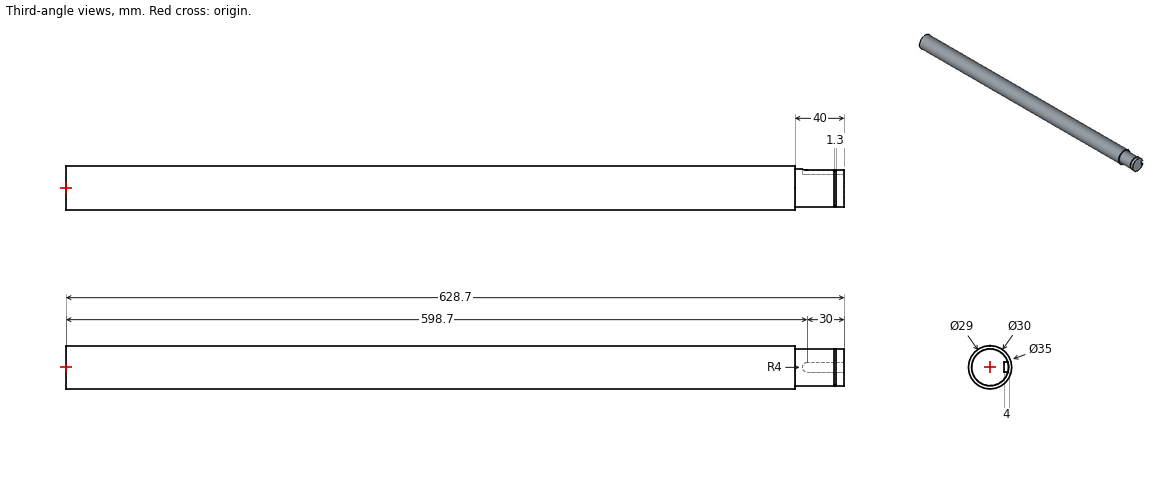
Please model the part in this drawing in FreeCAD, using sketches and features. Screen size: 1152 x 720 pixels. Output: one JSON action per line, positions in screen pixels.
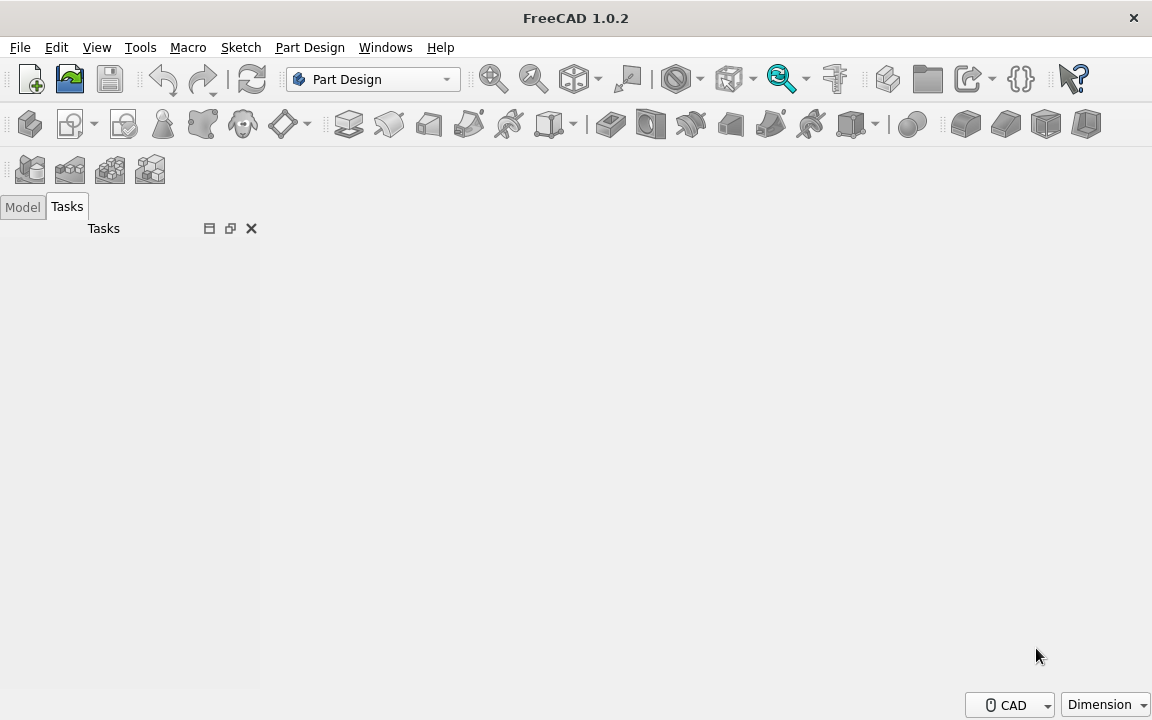
{"action": "left_click", "coordinate": [30, 80]}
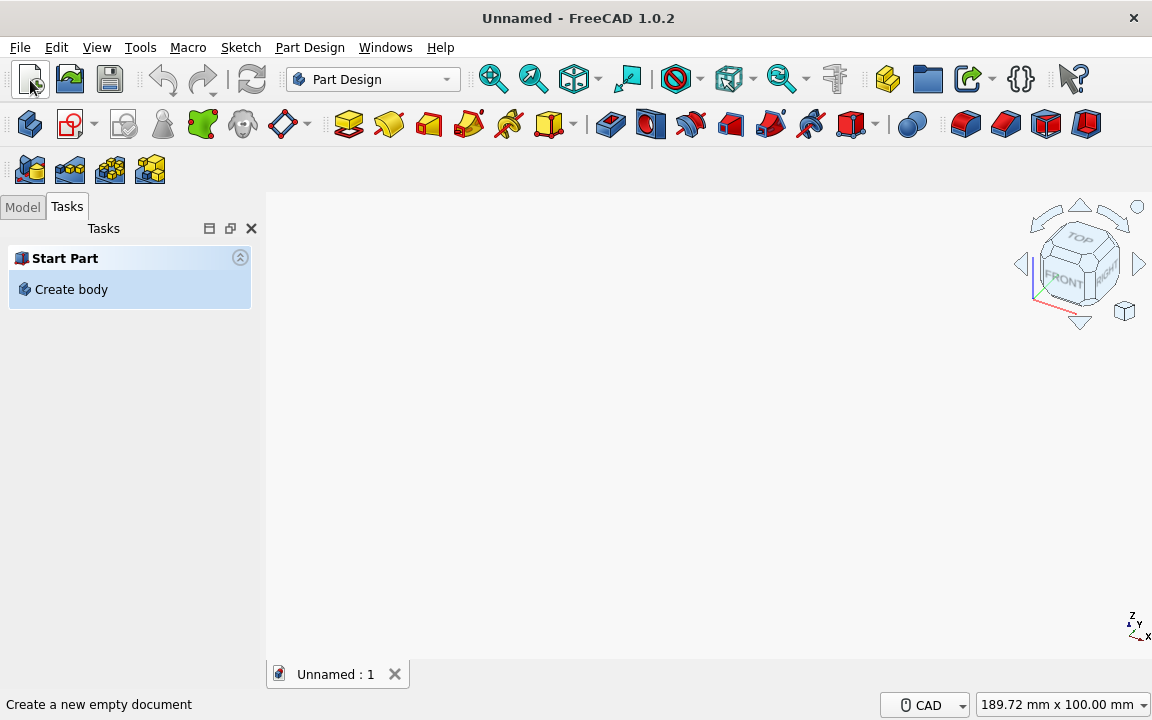
{"action": "left_click", "coordinate": [70, 124]}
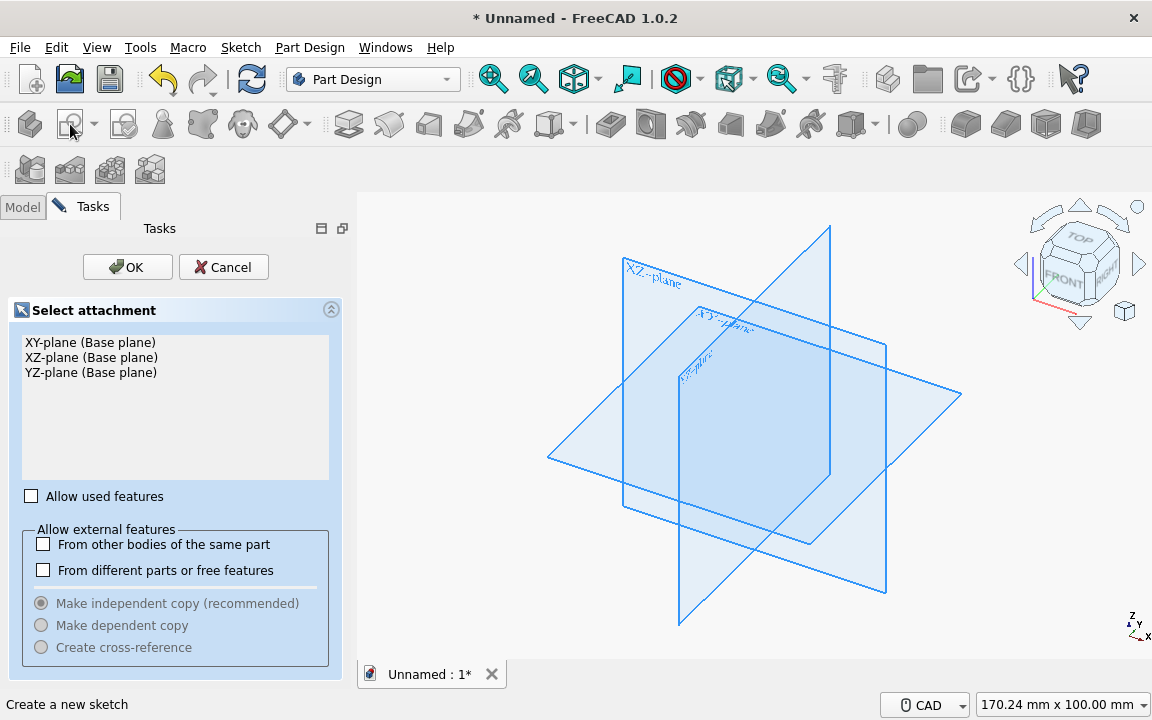
{"action": "left_click", "coordinate": [82, 372]}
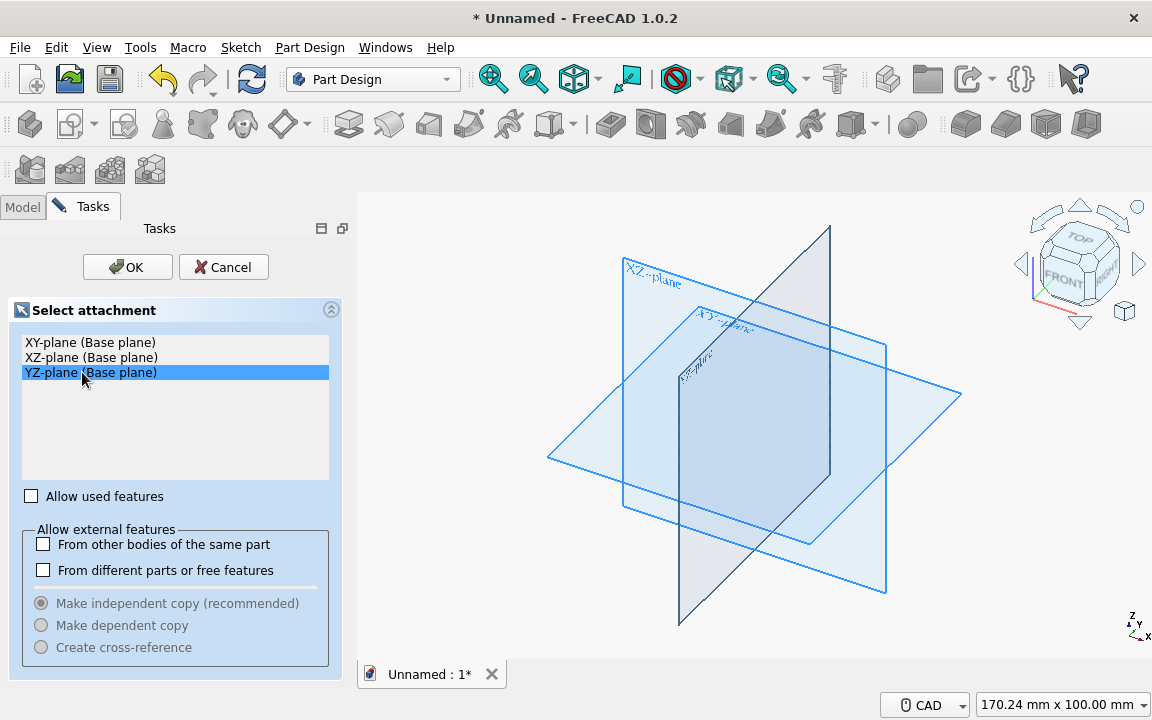
{"action": "left_click", "coordinate": [128, 267]}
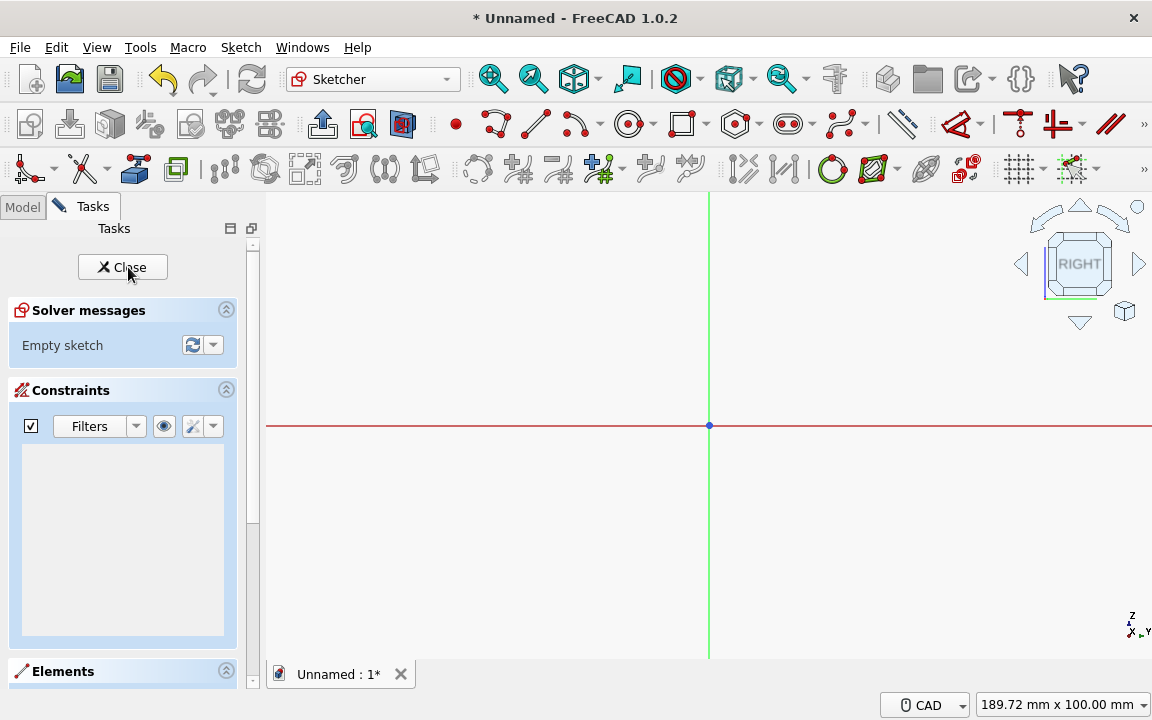
{"action": "scroll", "coordinate": [792, 426], "scroll_direction": "up", "scroll_amount": 3}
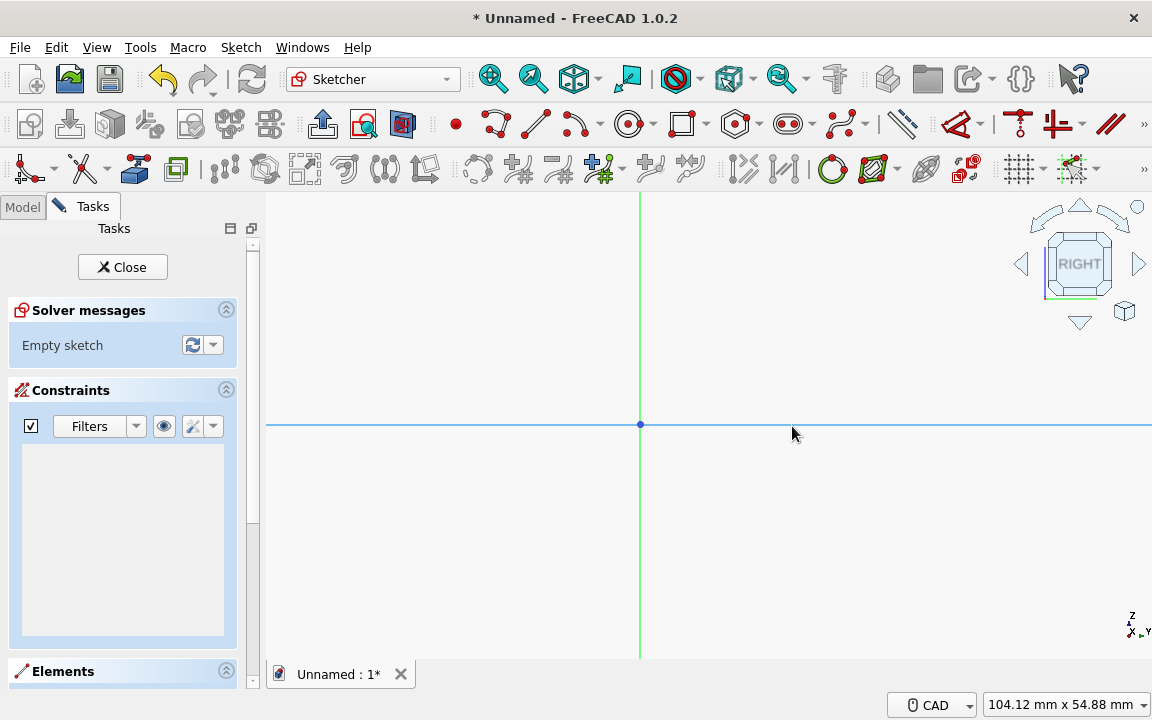
{"action": "left_click", "coordinate": [630, 124]}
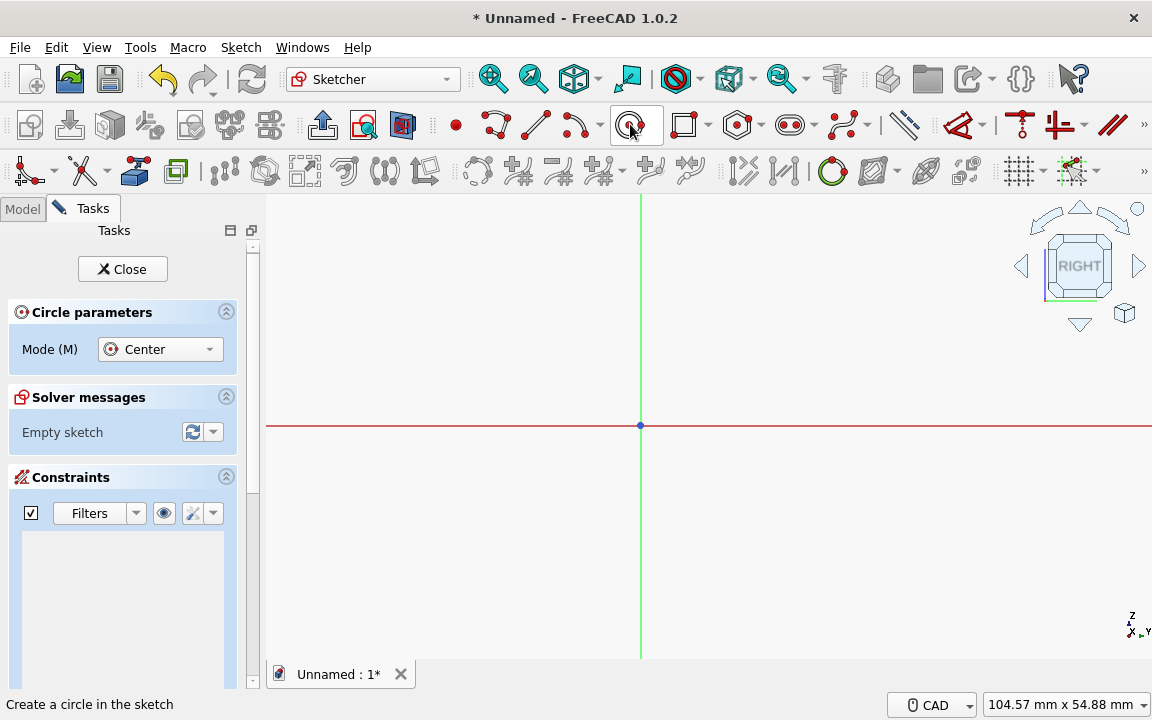
{"action": "left_click", "coordinate": [641, 426]}
{"action": "left_click", "coordinate": [745, 321]}
{"action": "key", "text": "Escape"}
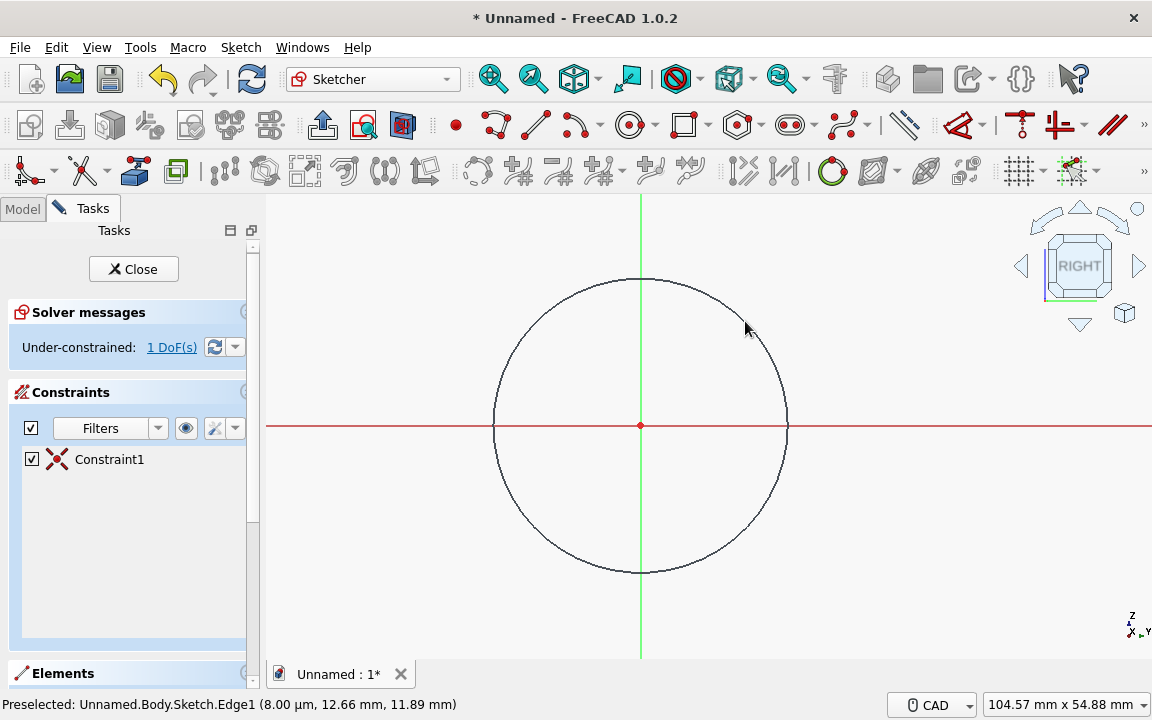
{"action": "left_click", "coordinate": [958, 126]}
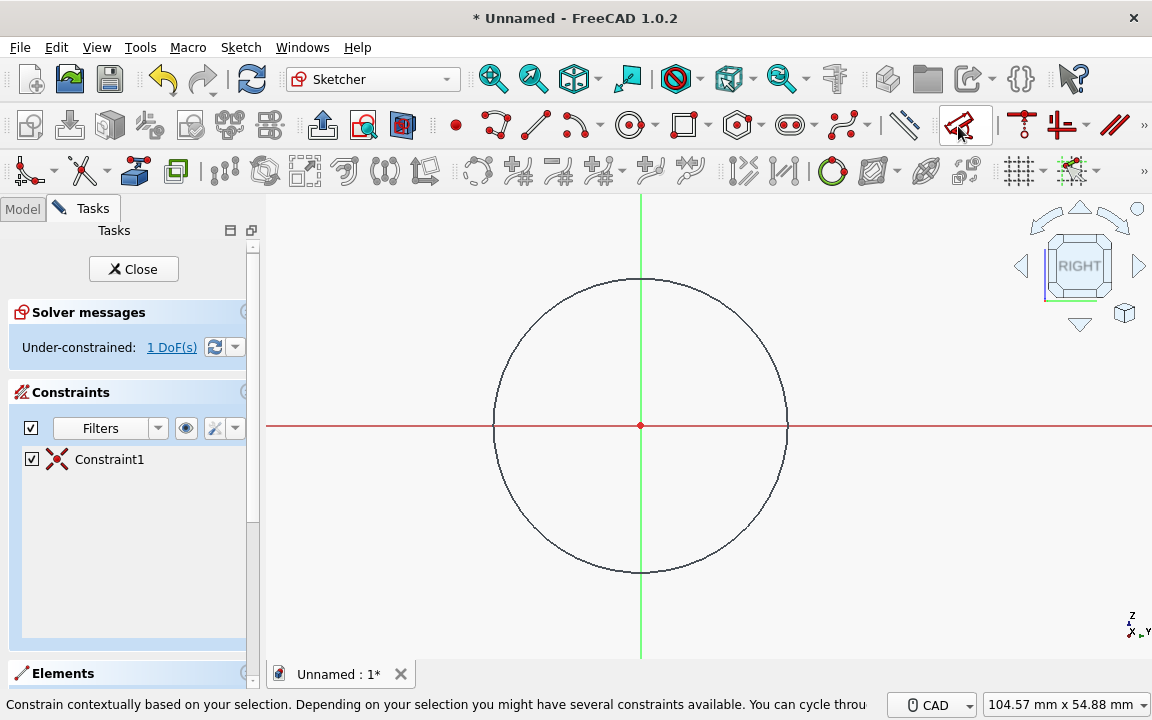
{"action": "left_click", "coordinate": [744, 321]}
{"action": "left_click", "coordinate": [766, 298]}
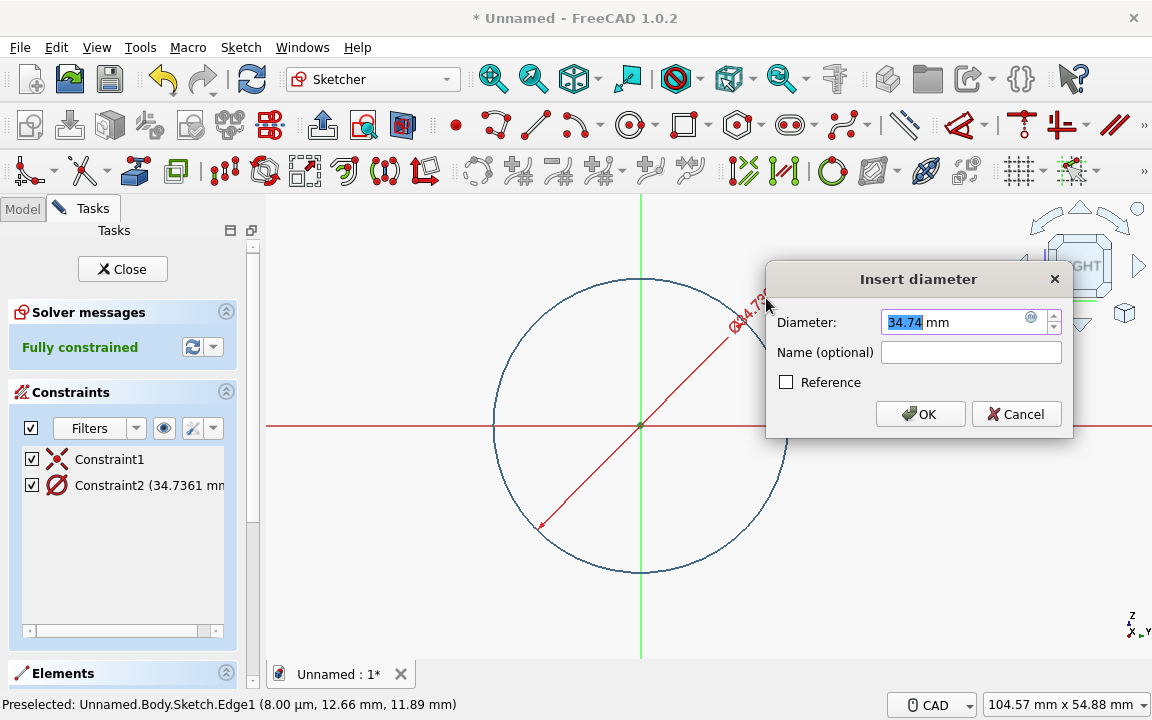
{"action": "type", "text": "35"}
{"action": "key", "text": "Return"}
{"action": "key", "text": "Escape"}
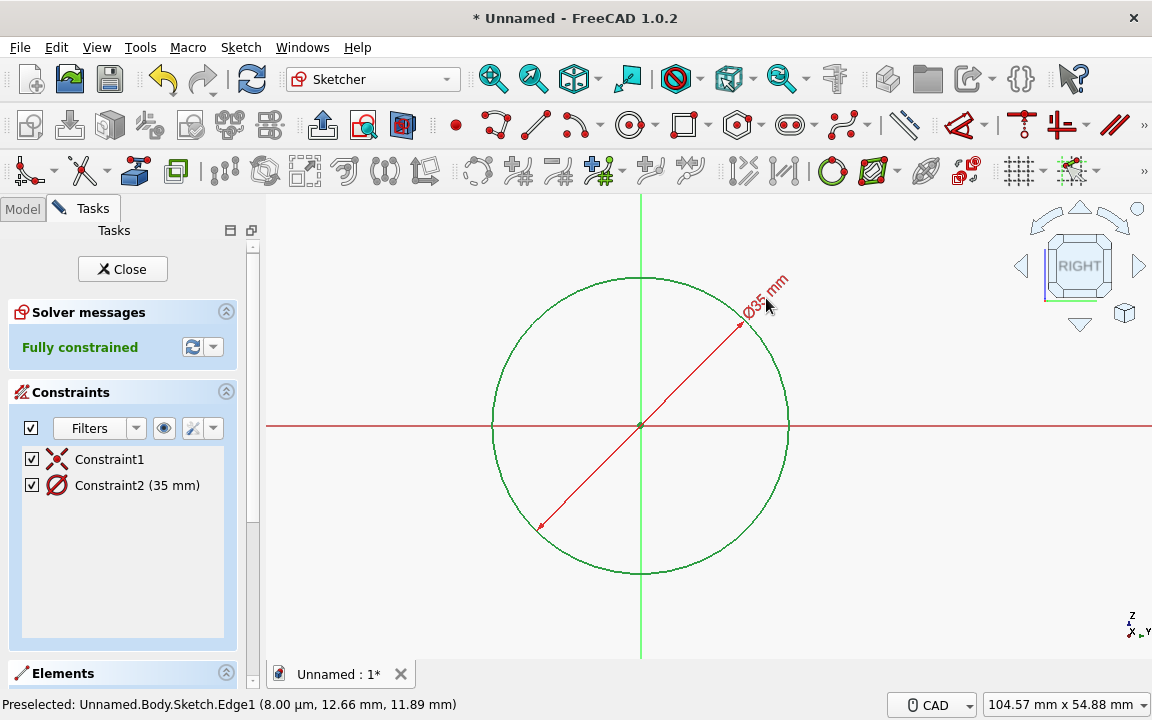
{"action": "left_click", "coordinate": [123, 269]}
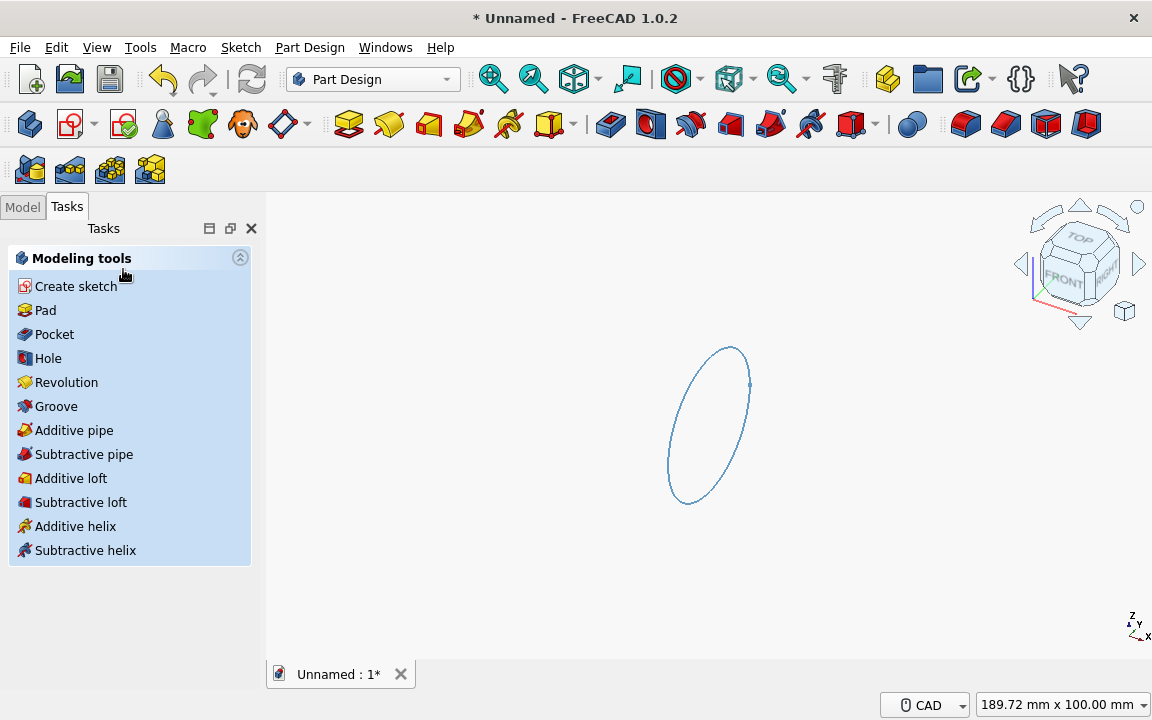
{"action": "left_click", "coordinate": [350, 124]}